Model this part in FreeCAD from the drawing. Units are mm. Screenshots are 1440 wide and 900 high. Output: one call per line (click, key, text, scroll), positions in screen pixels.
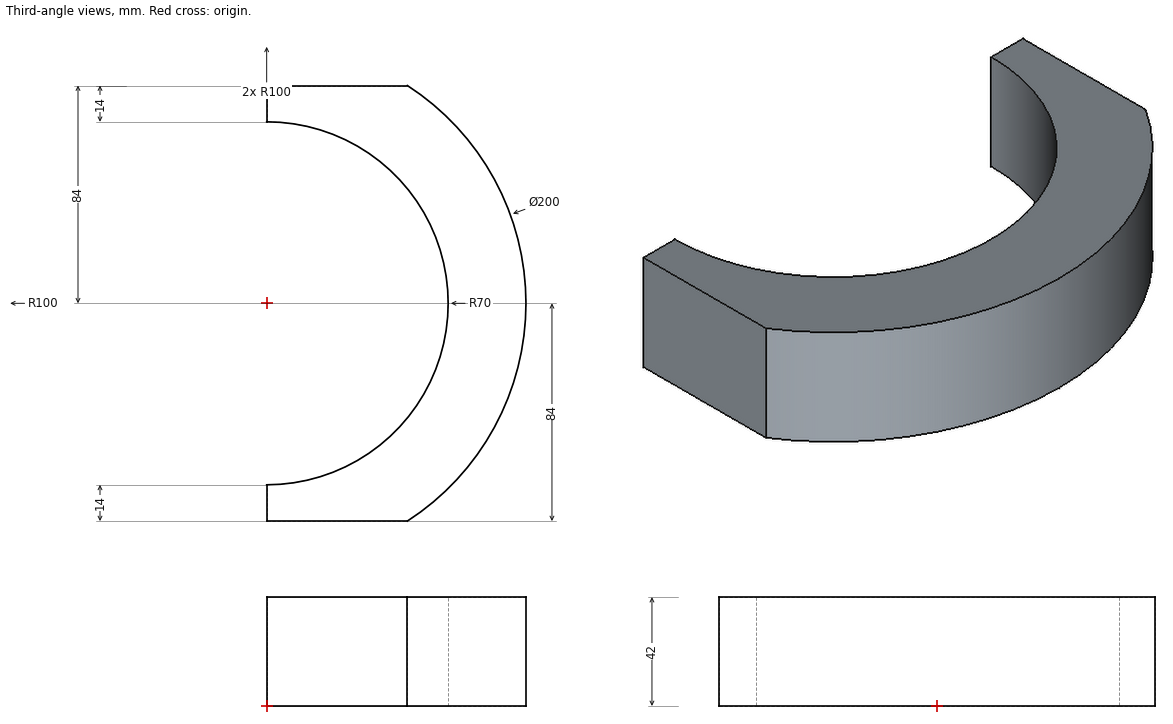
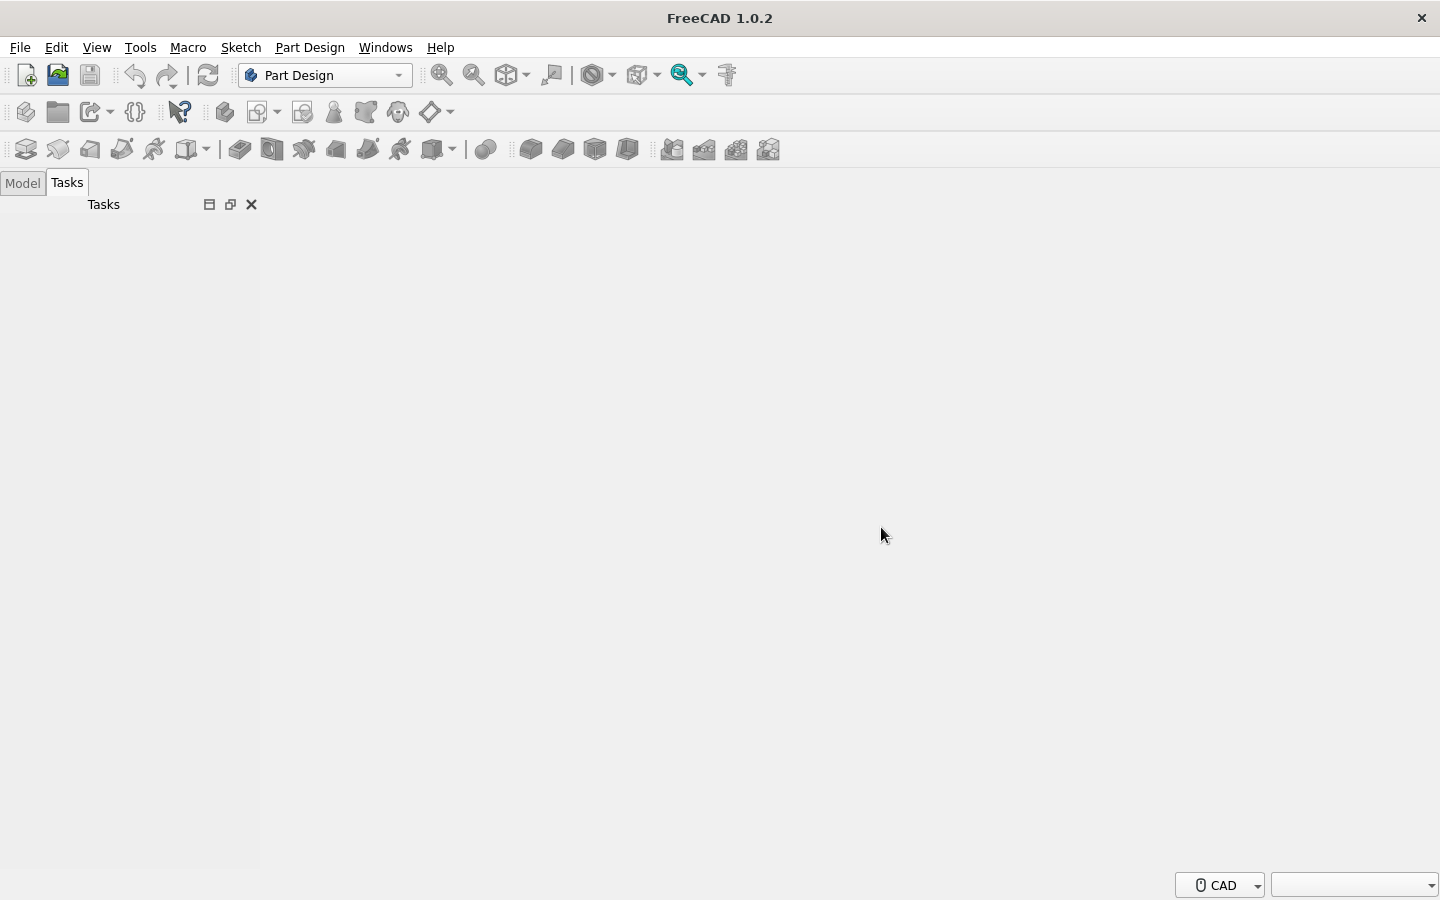
key(ctrl+n)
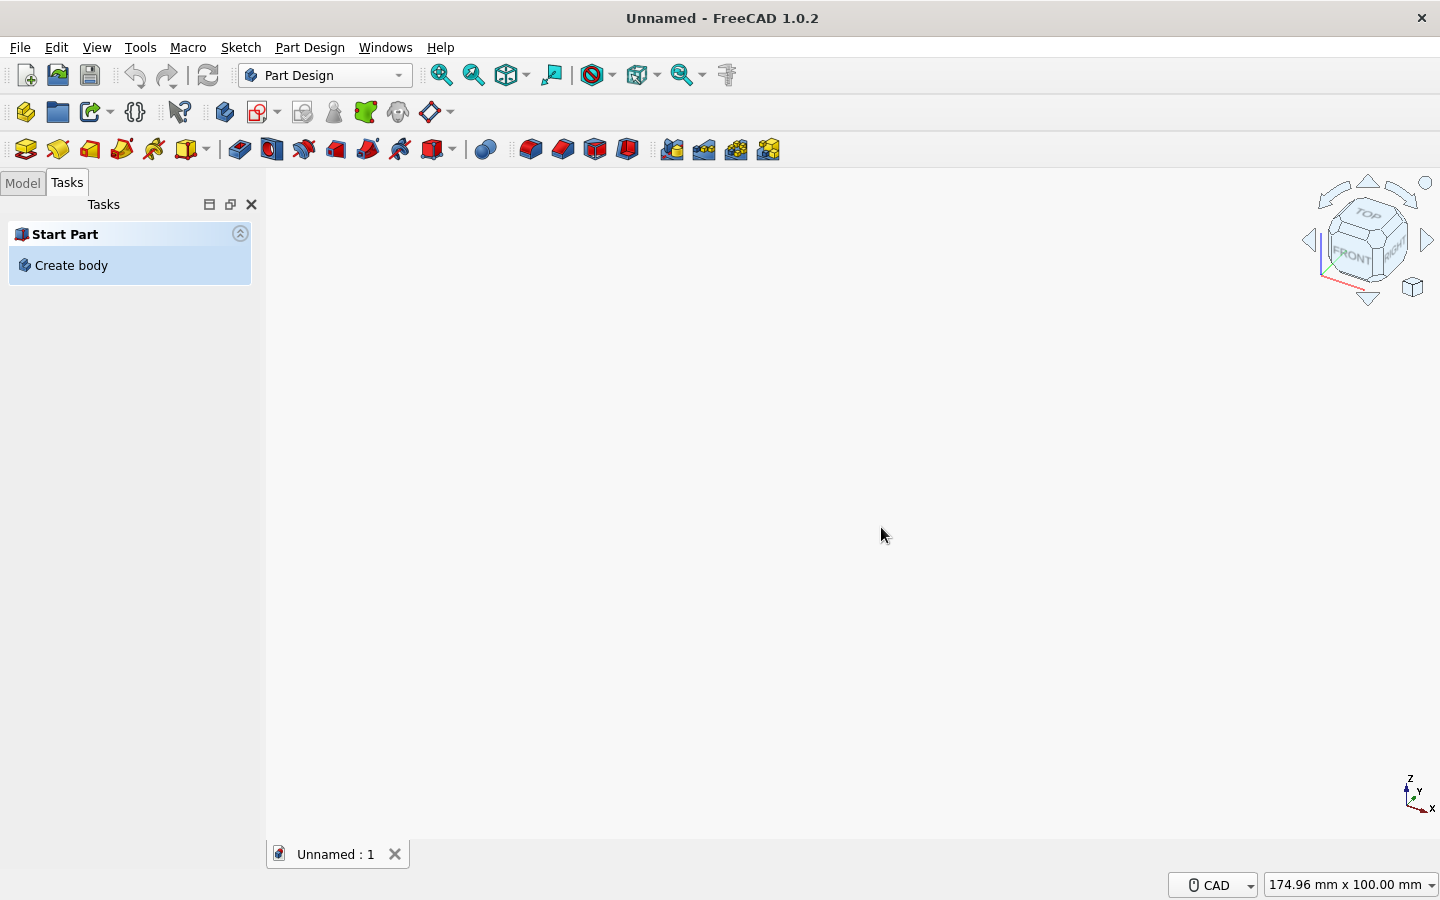
click(258, 112)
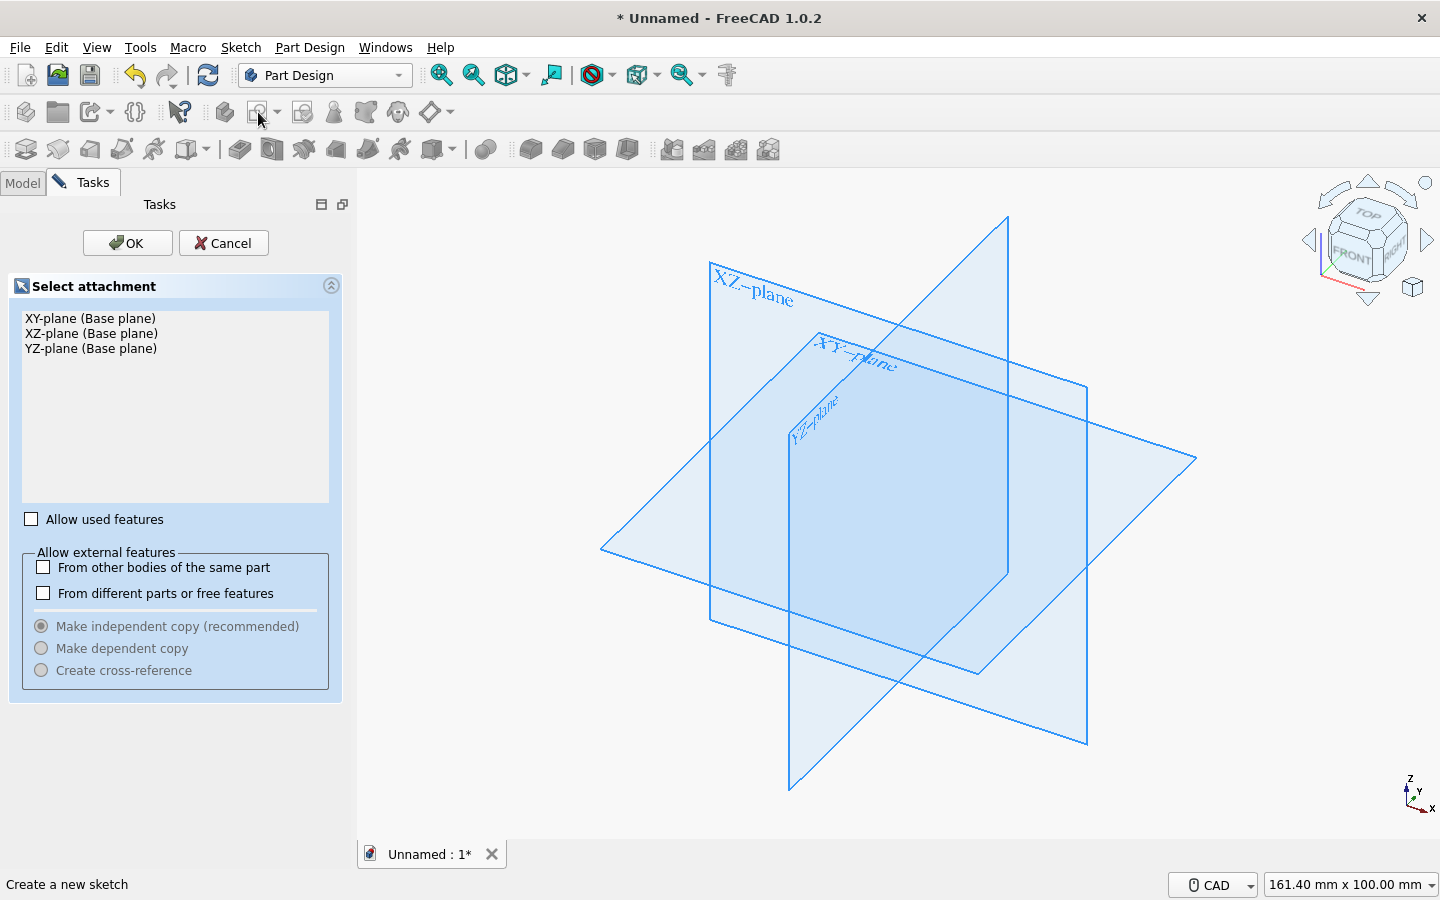
click(82, 318)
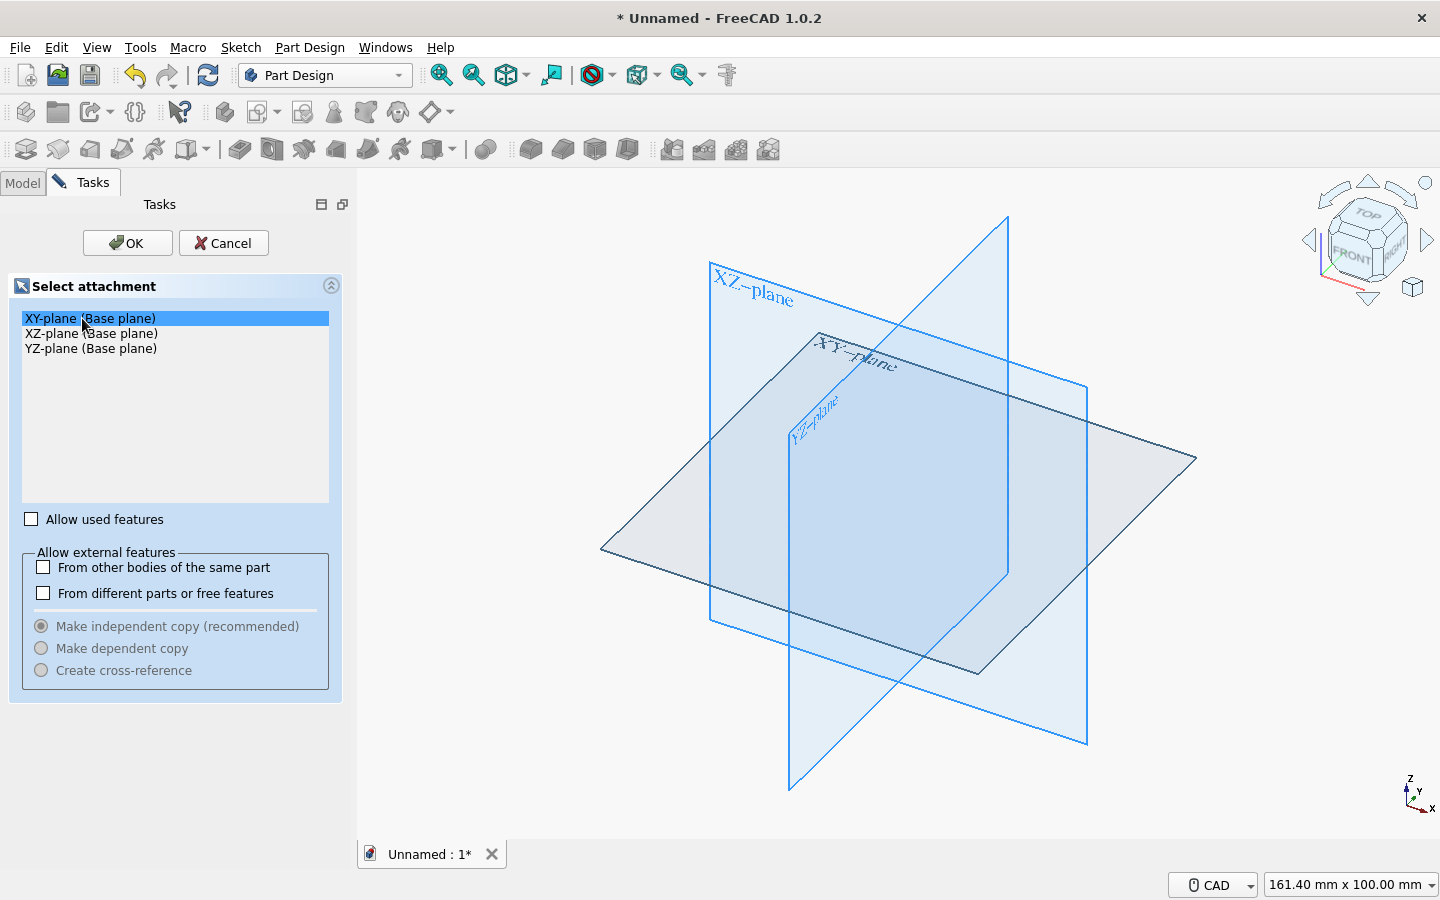
click(128, 243)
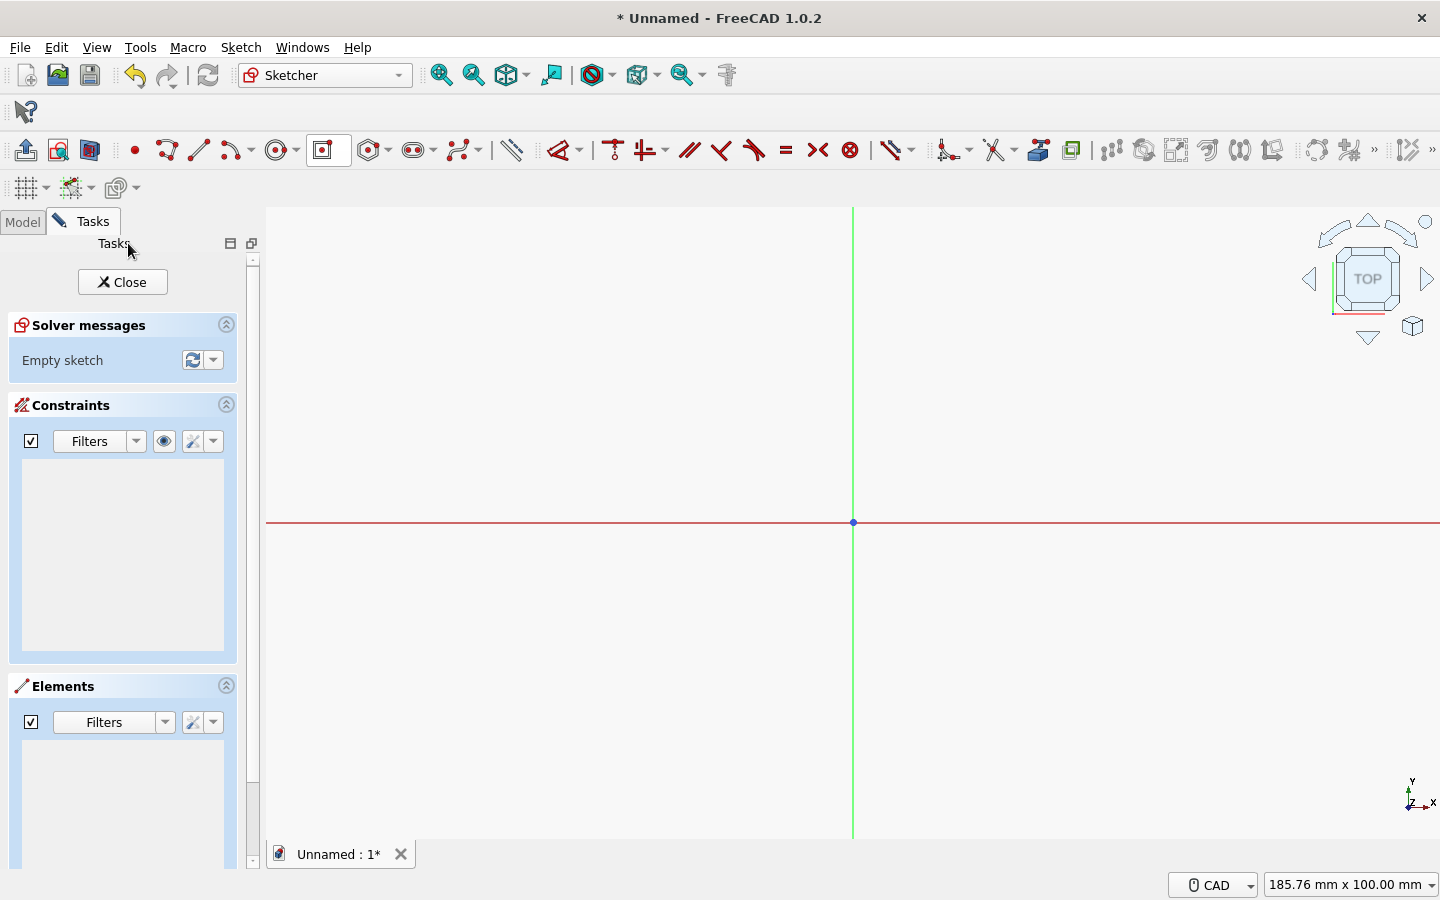
scroll(755, 523, down, 6)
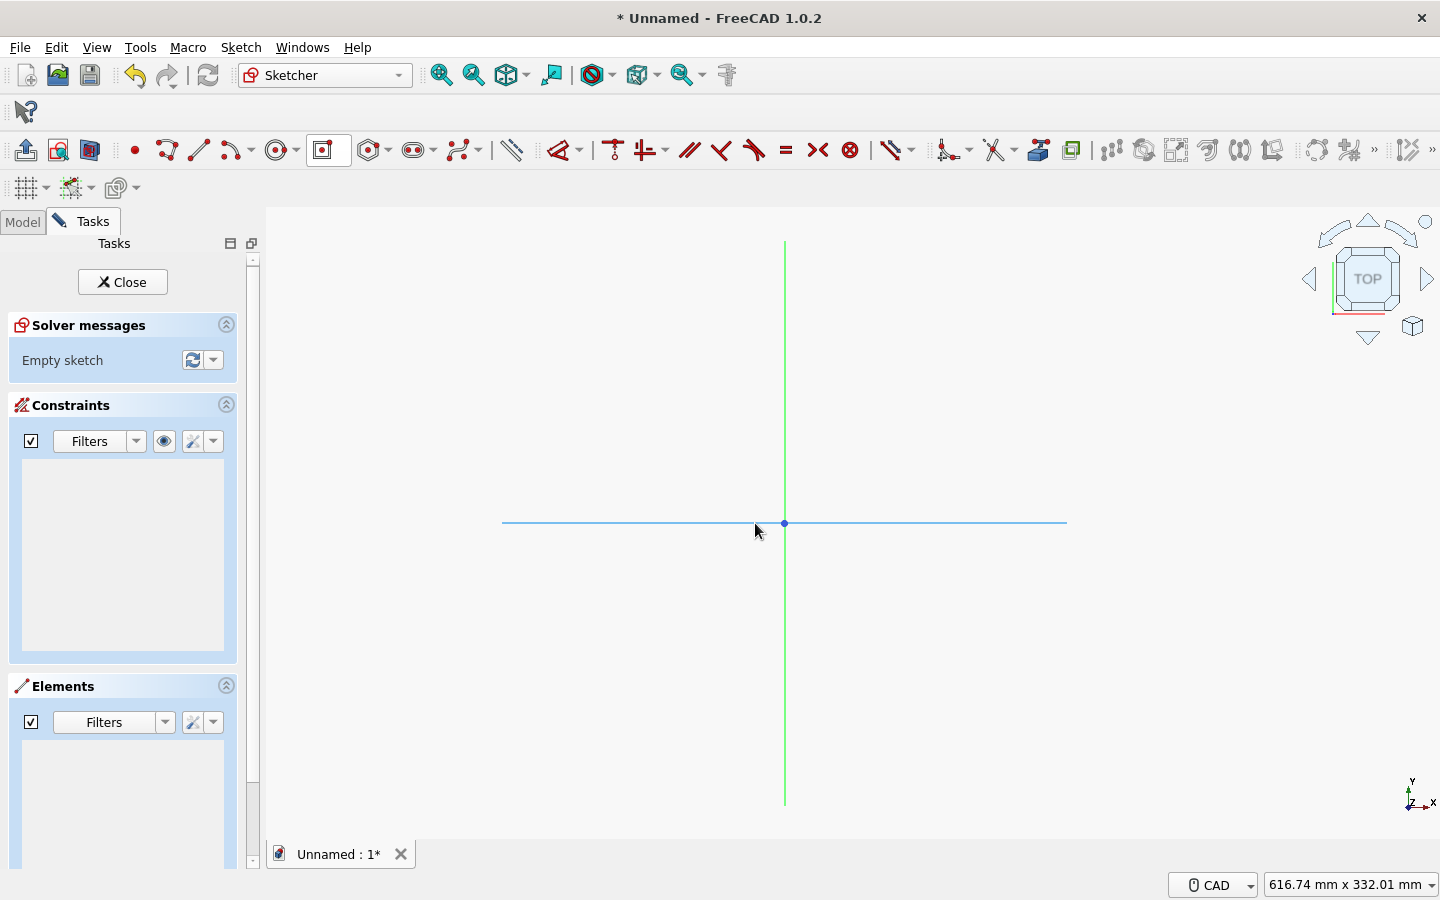
click(276, 150)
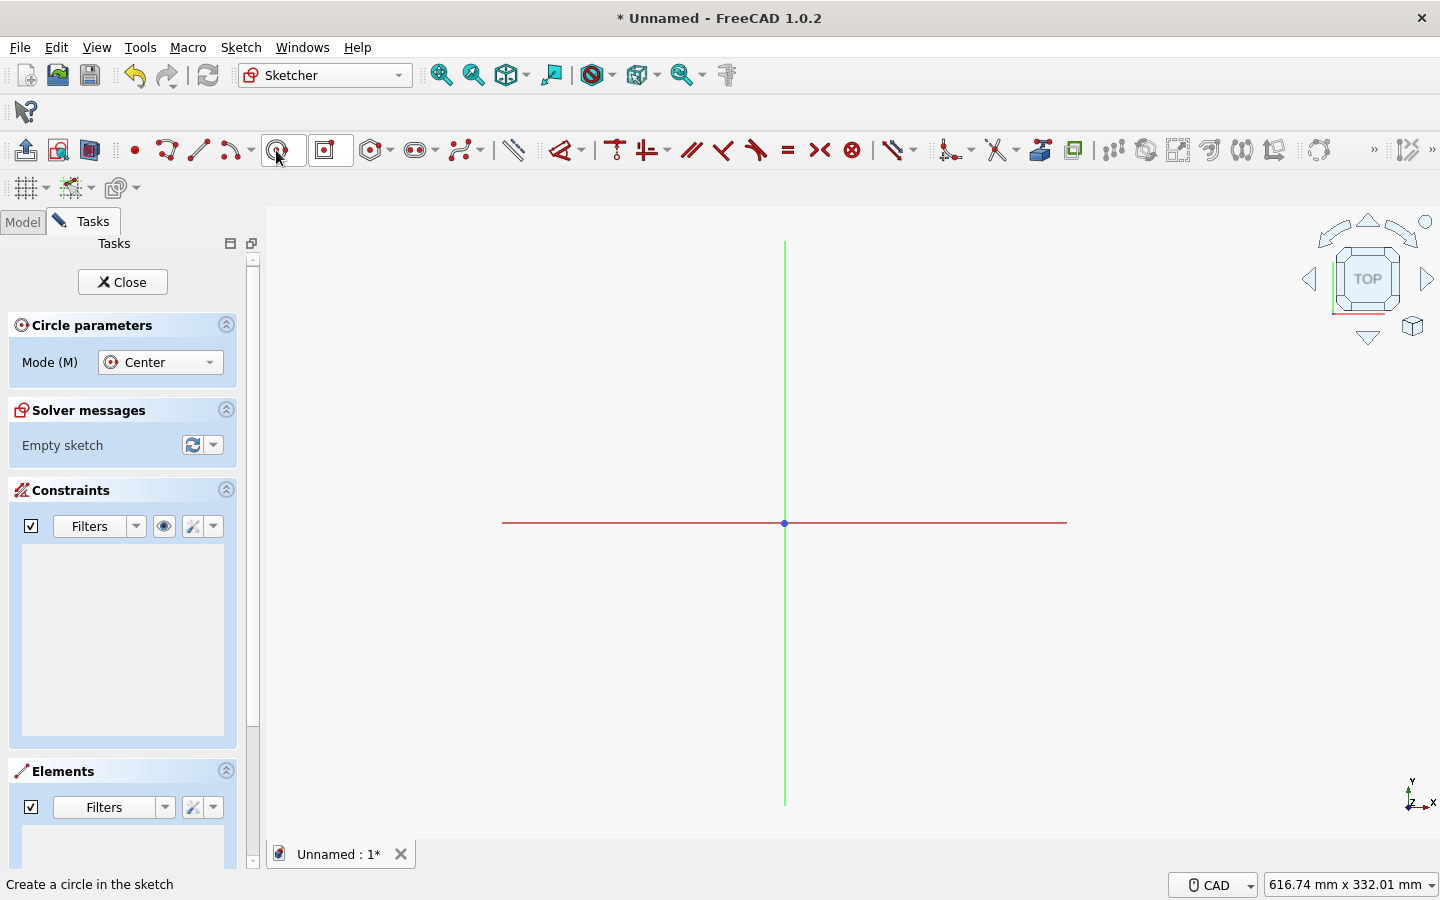
click(785, 523)
move(919, 389)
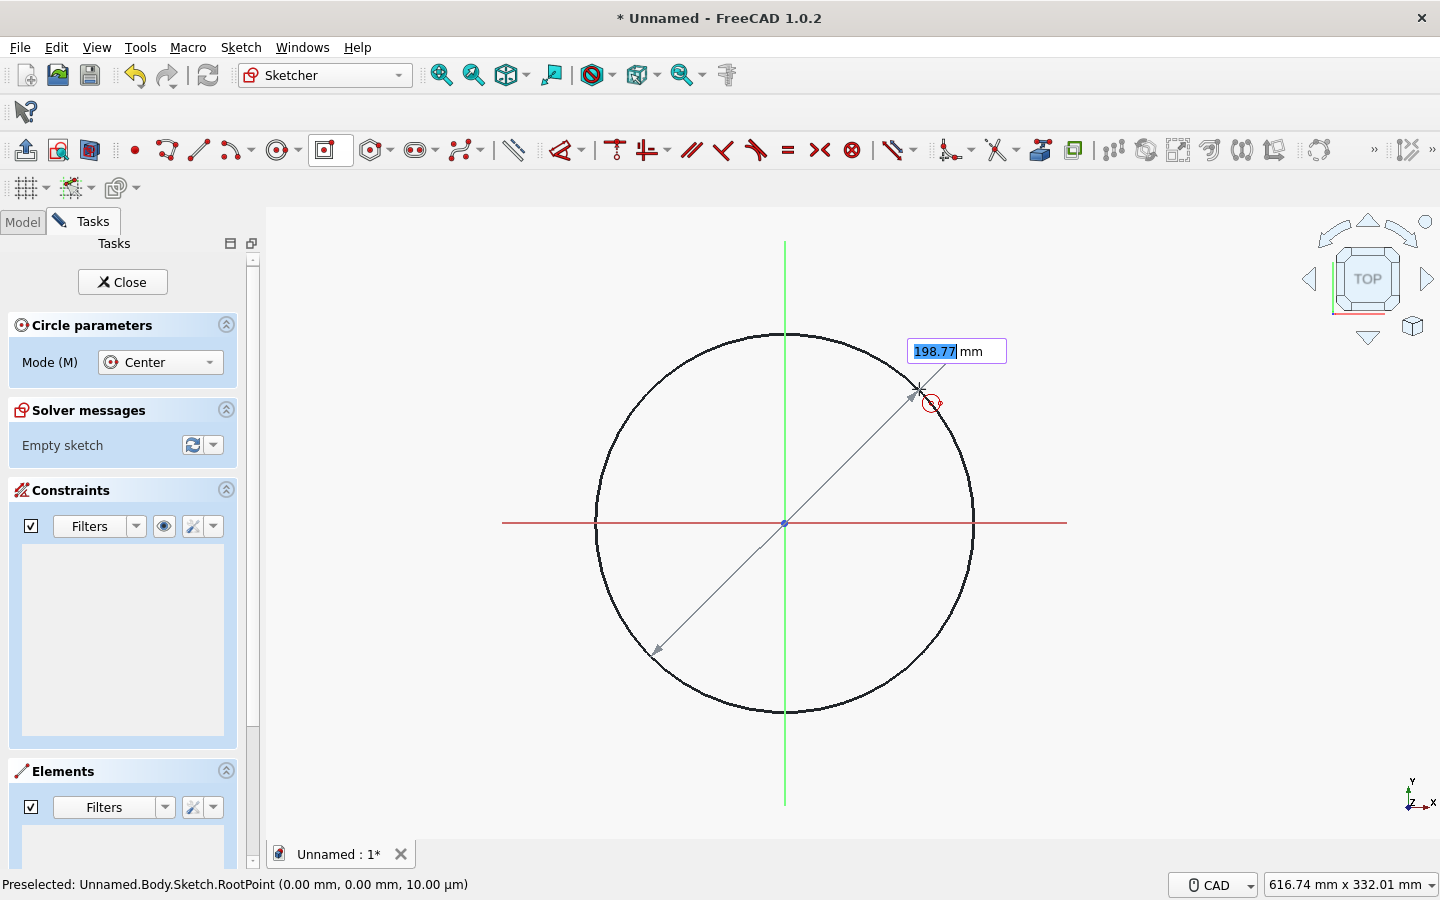
text(200)
key(Return)
key(Escape)